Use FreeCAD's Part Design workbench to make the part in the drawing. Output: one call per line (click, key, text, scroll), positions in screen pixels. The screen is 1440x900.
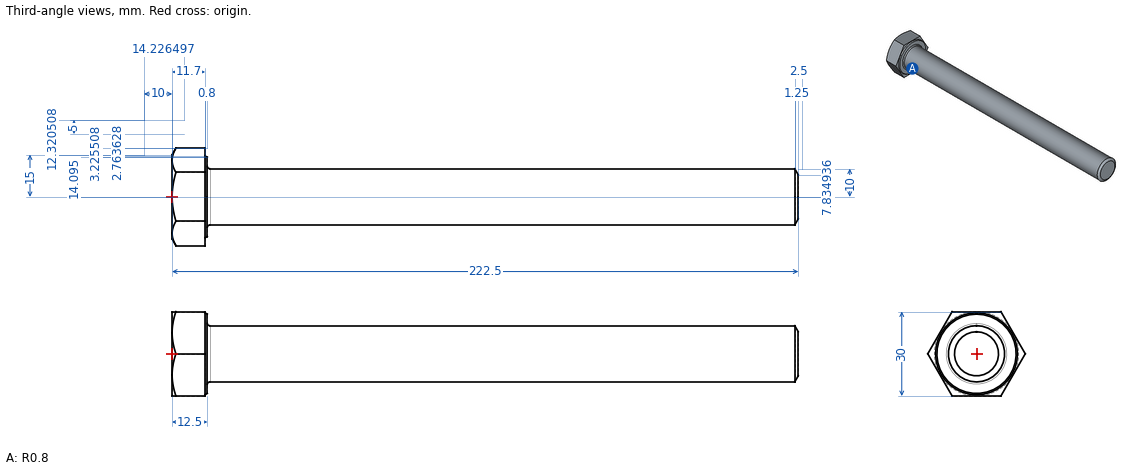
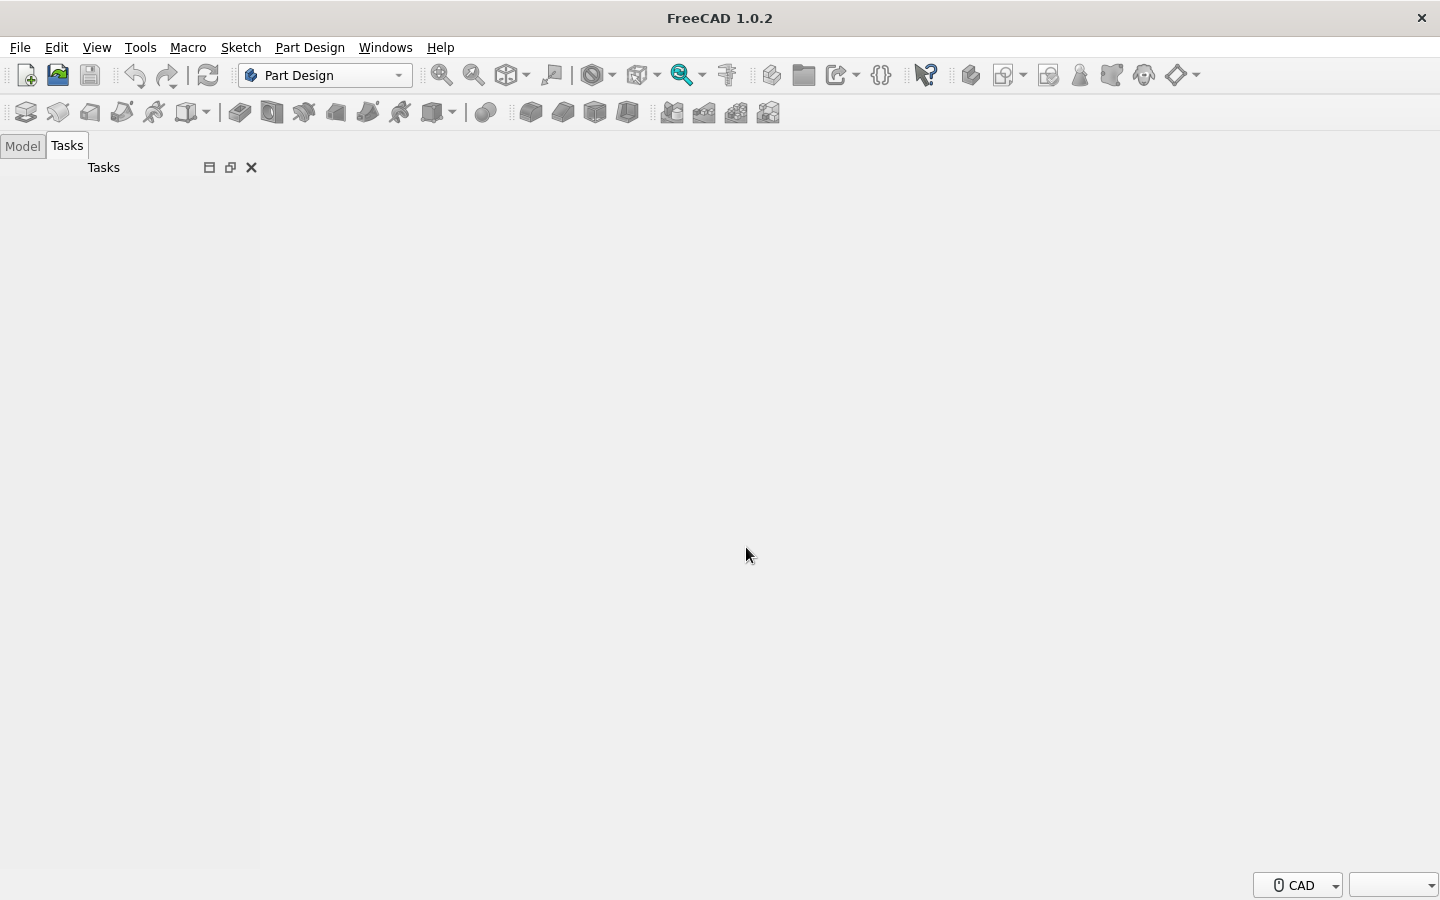
click(26, 76)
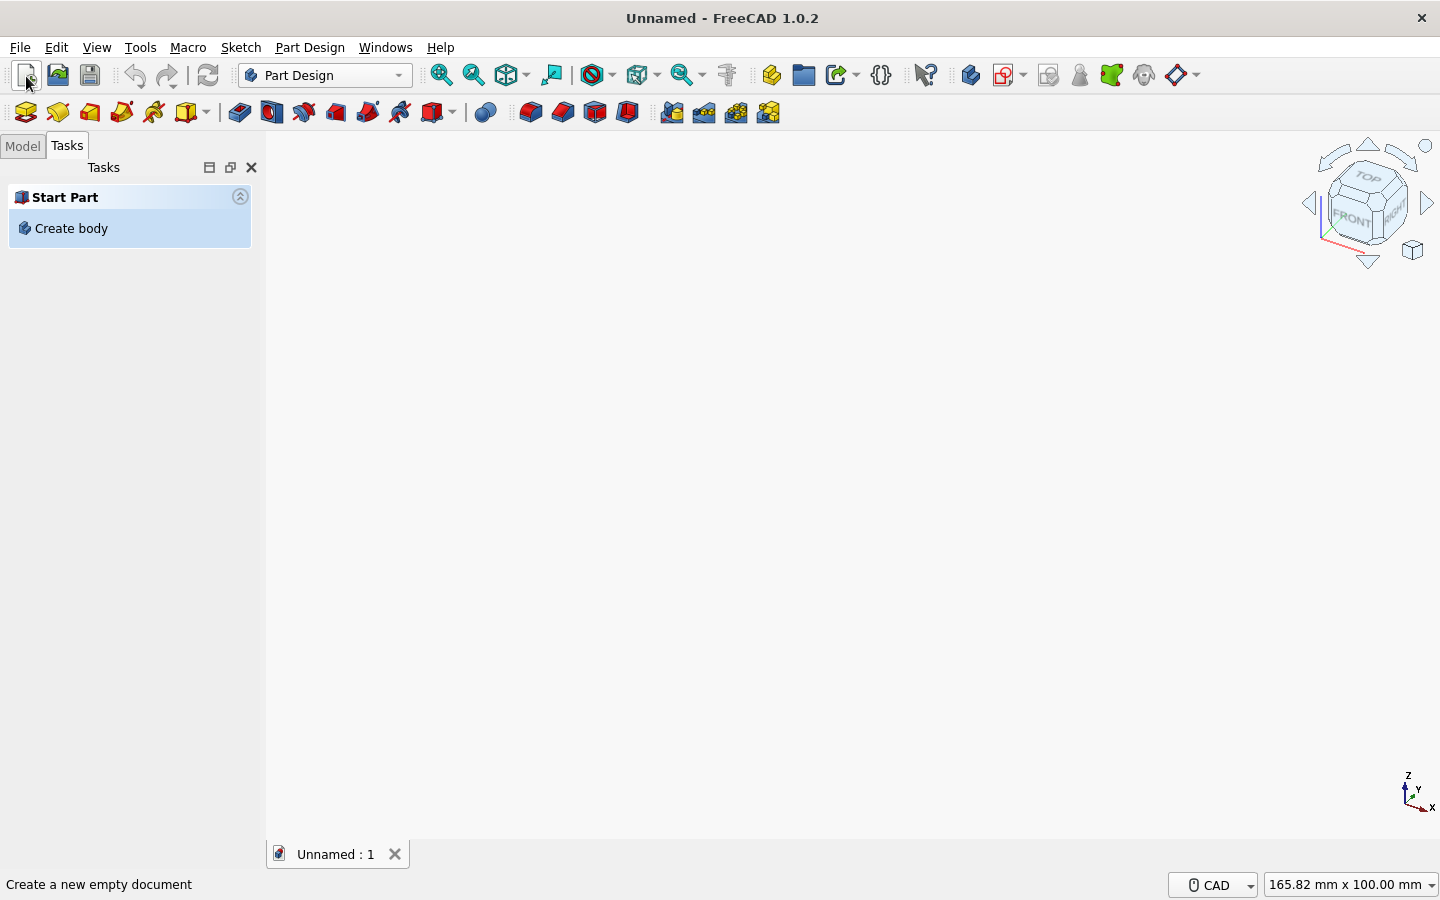
click(1004, 76)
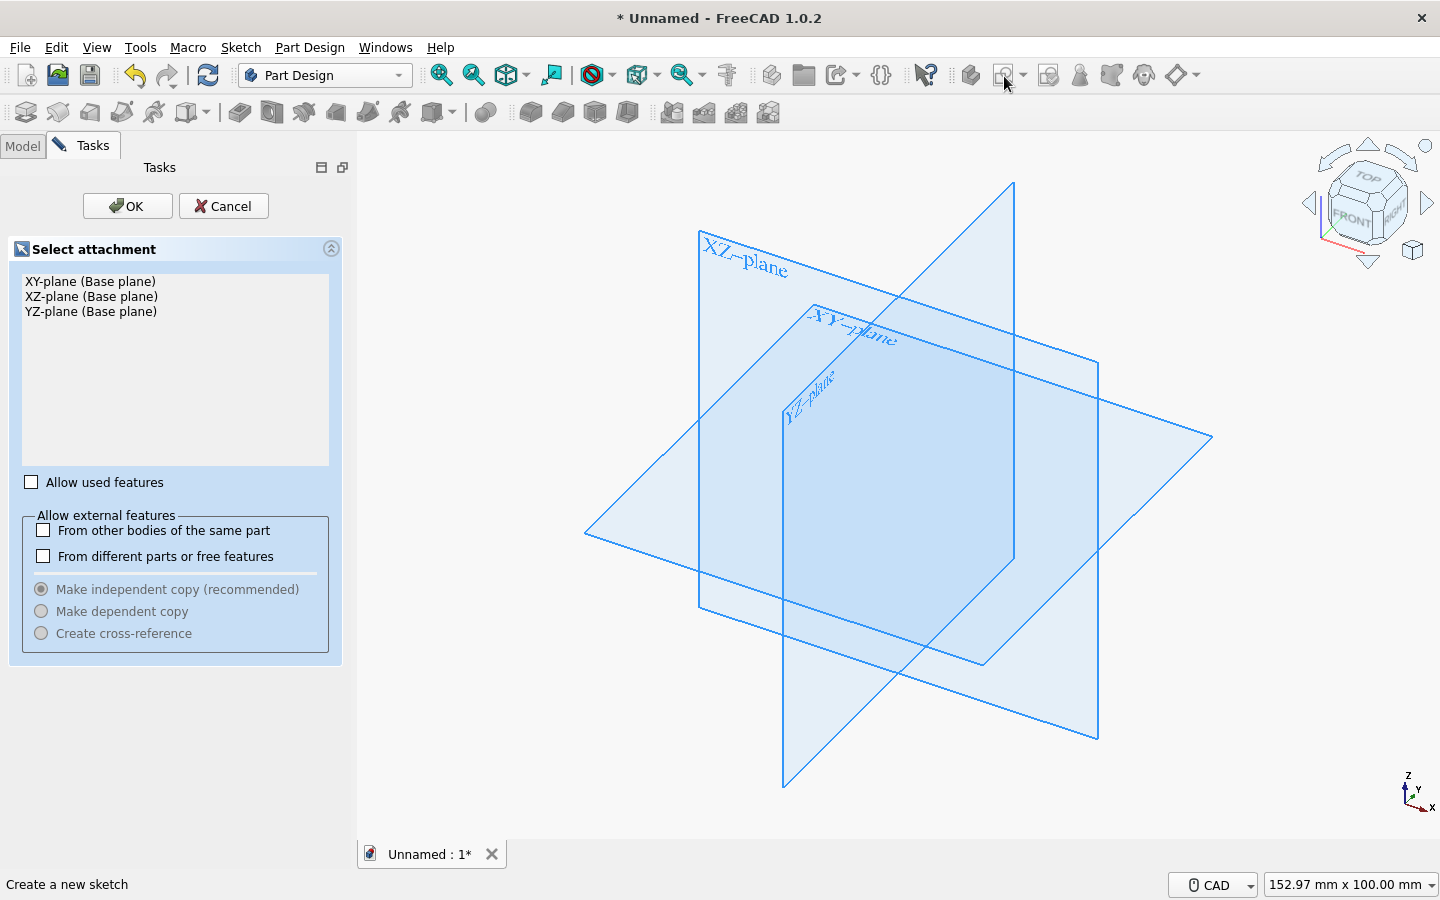
click(82, 312)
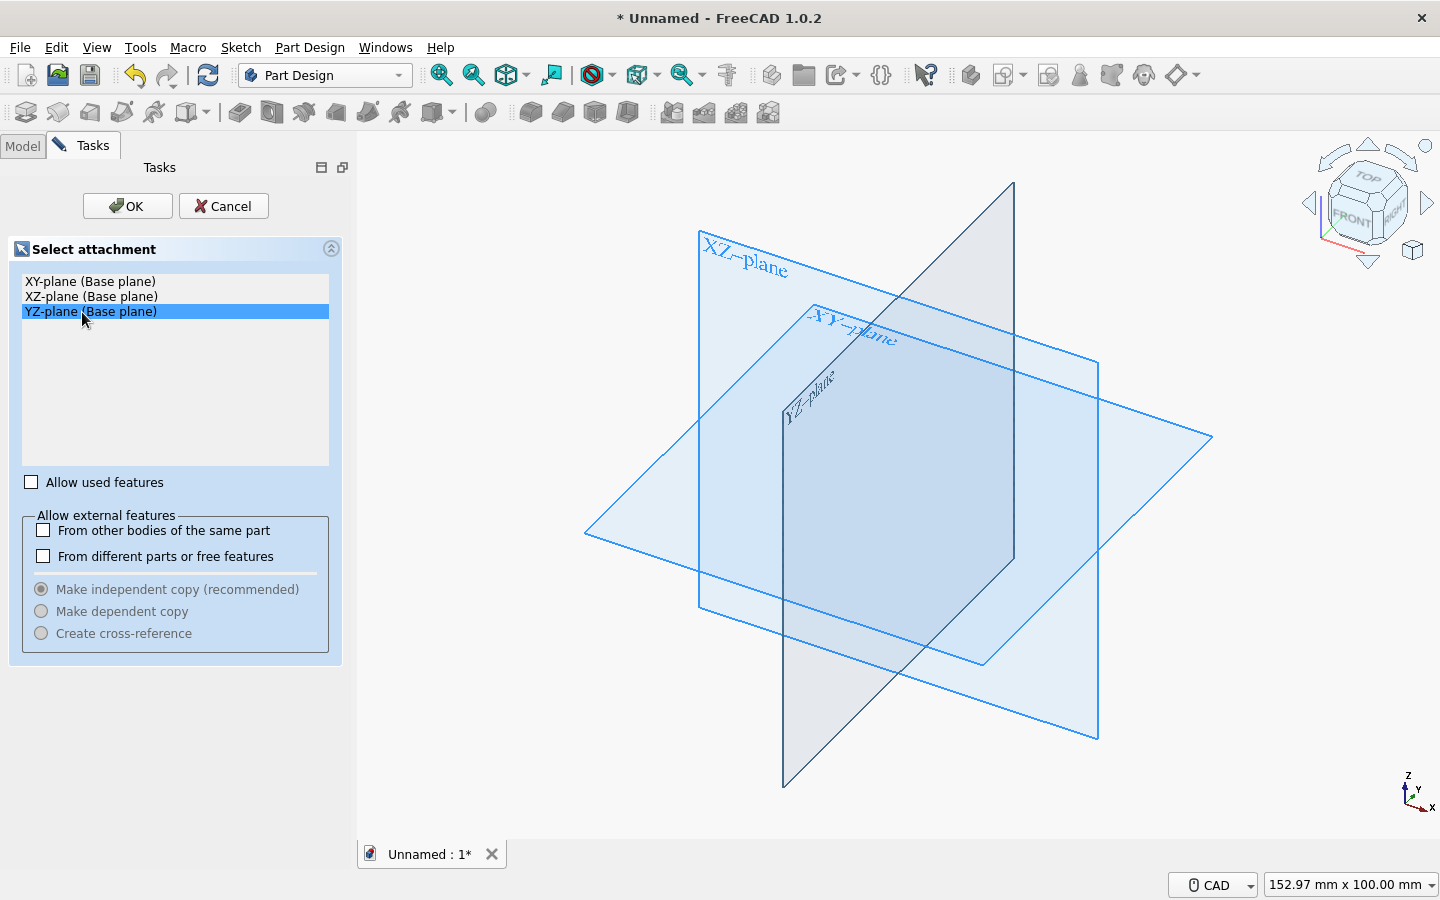
click(128, 206)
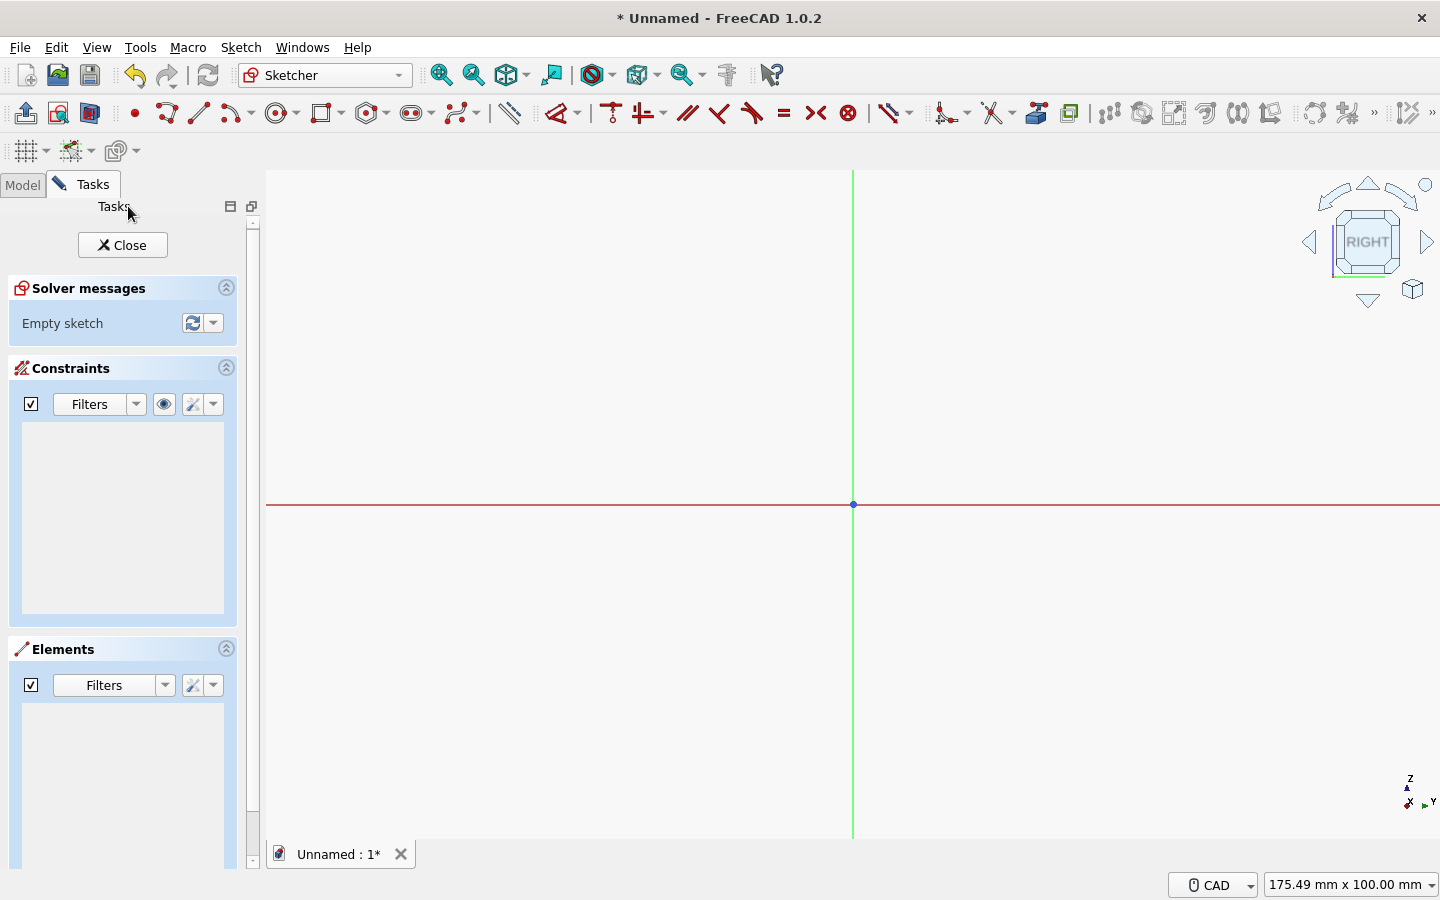
scroll(909, 504, up, 4)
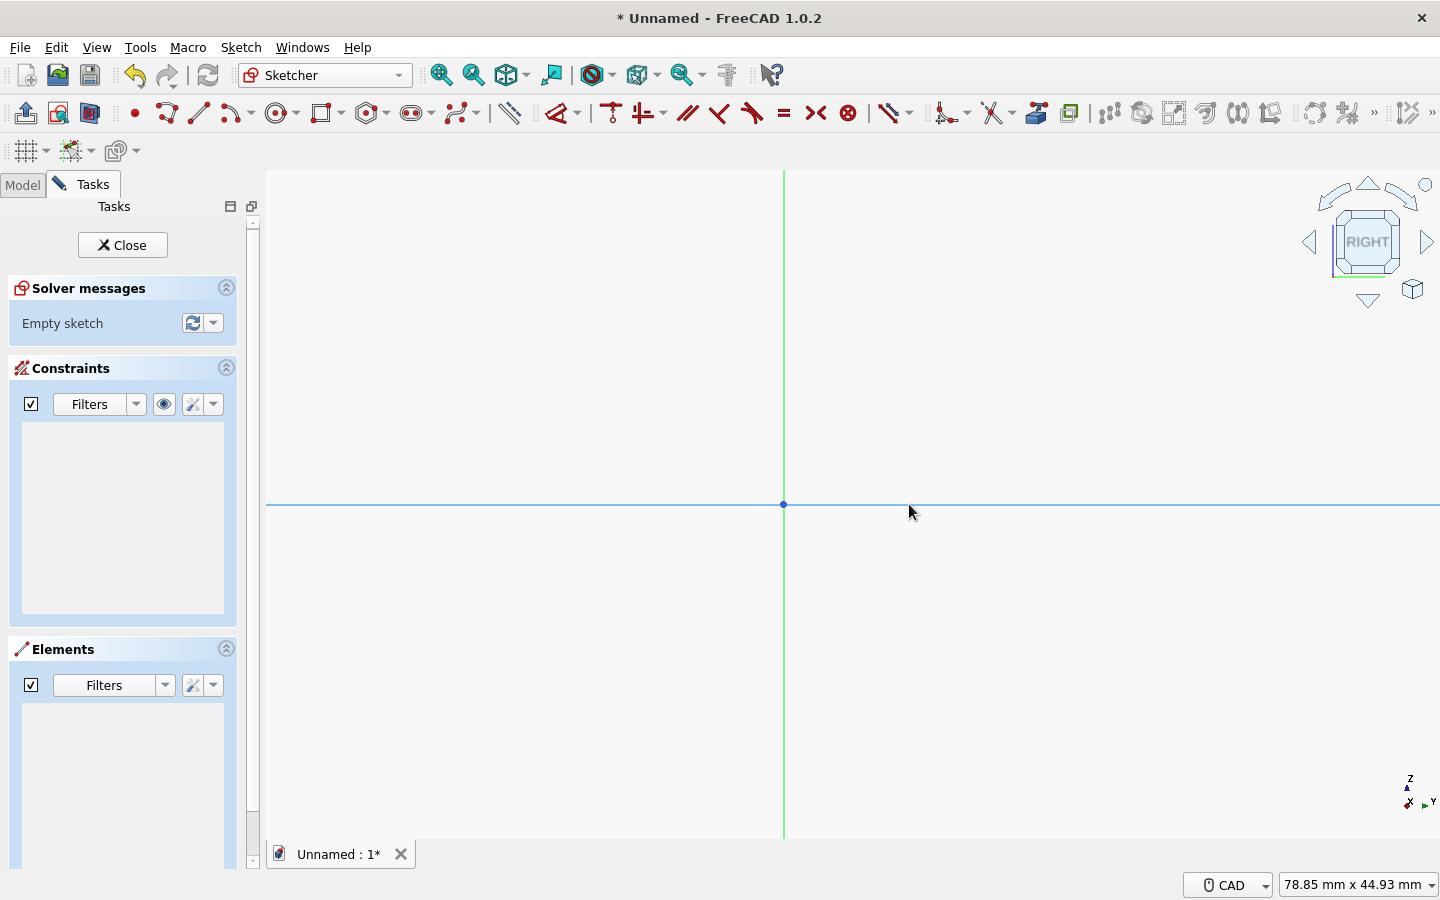
click(366, 114)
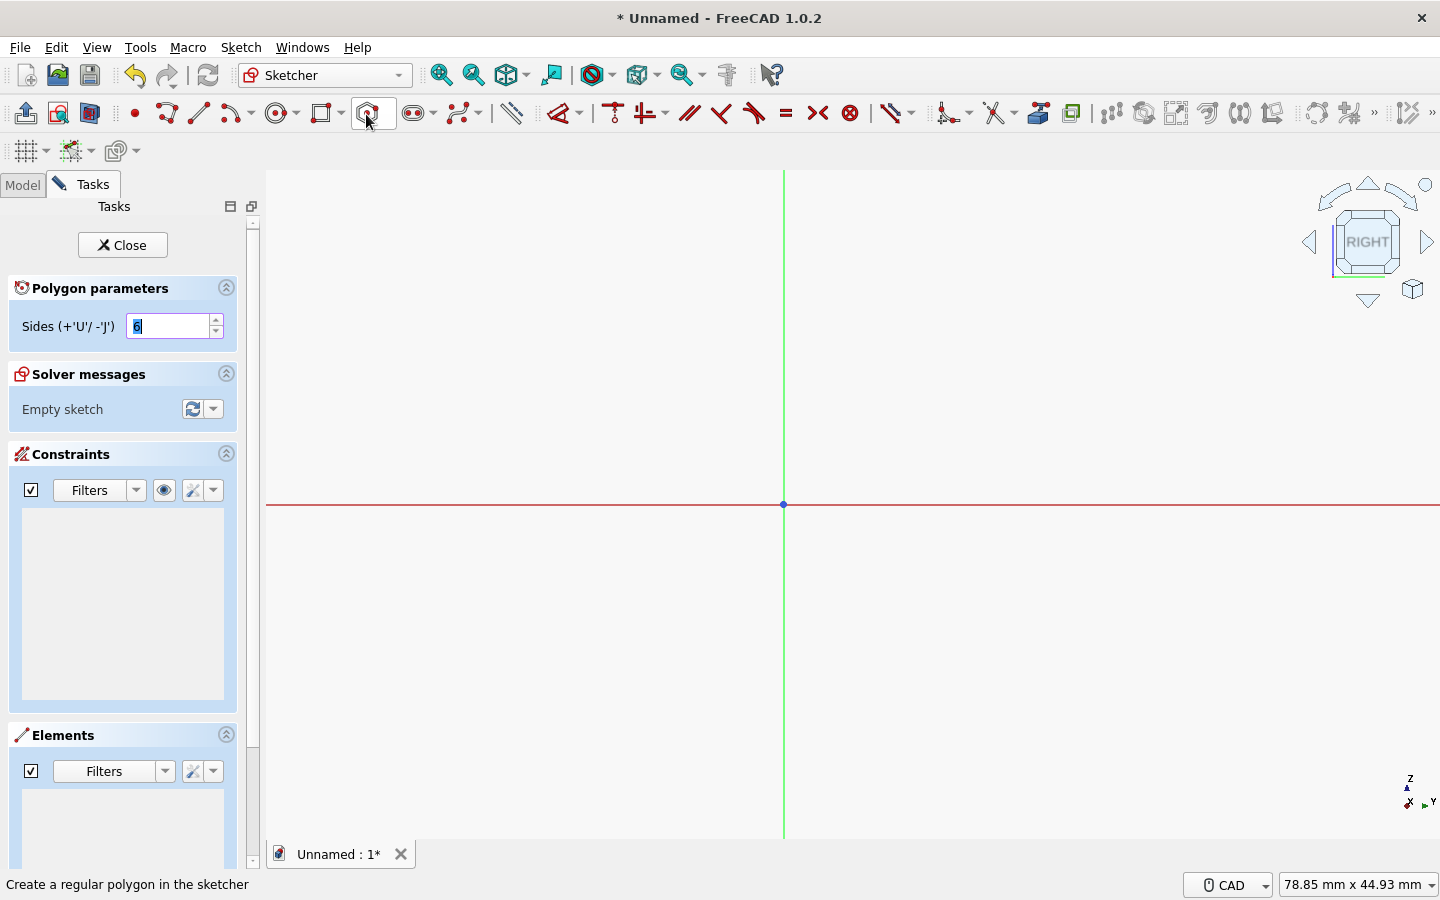
click(784, 504)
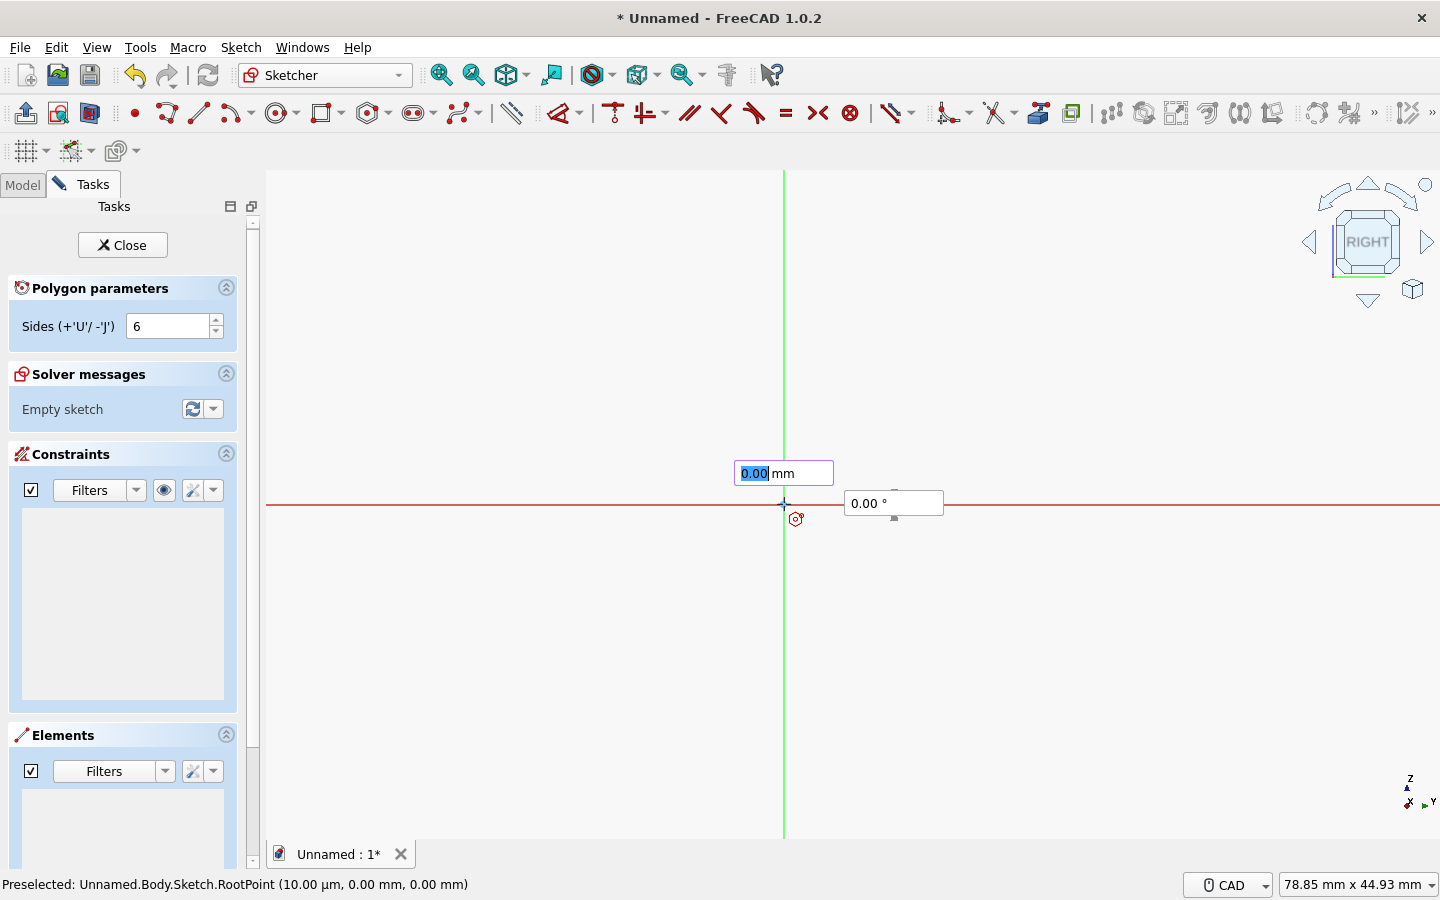
click(1042, 504)
right_click(1042, 504)